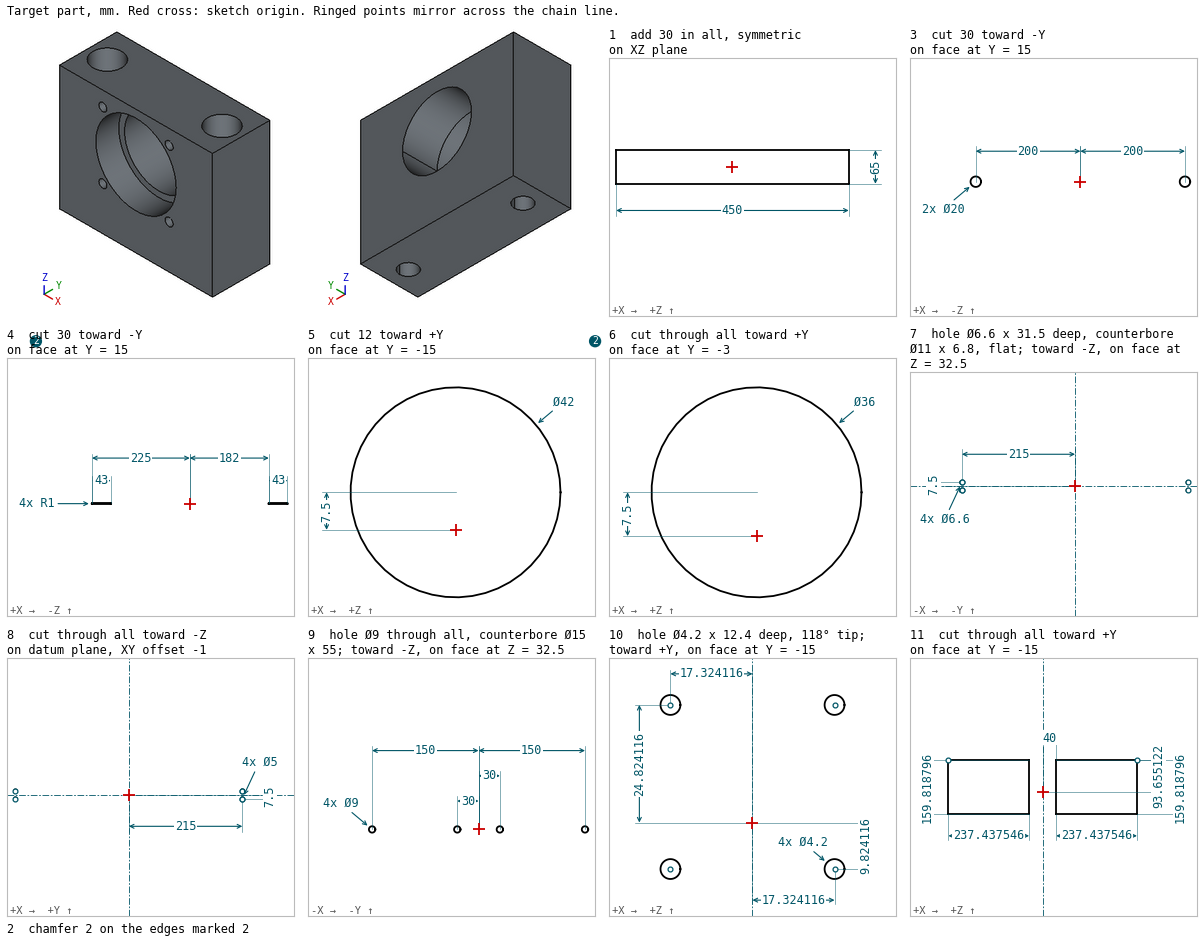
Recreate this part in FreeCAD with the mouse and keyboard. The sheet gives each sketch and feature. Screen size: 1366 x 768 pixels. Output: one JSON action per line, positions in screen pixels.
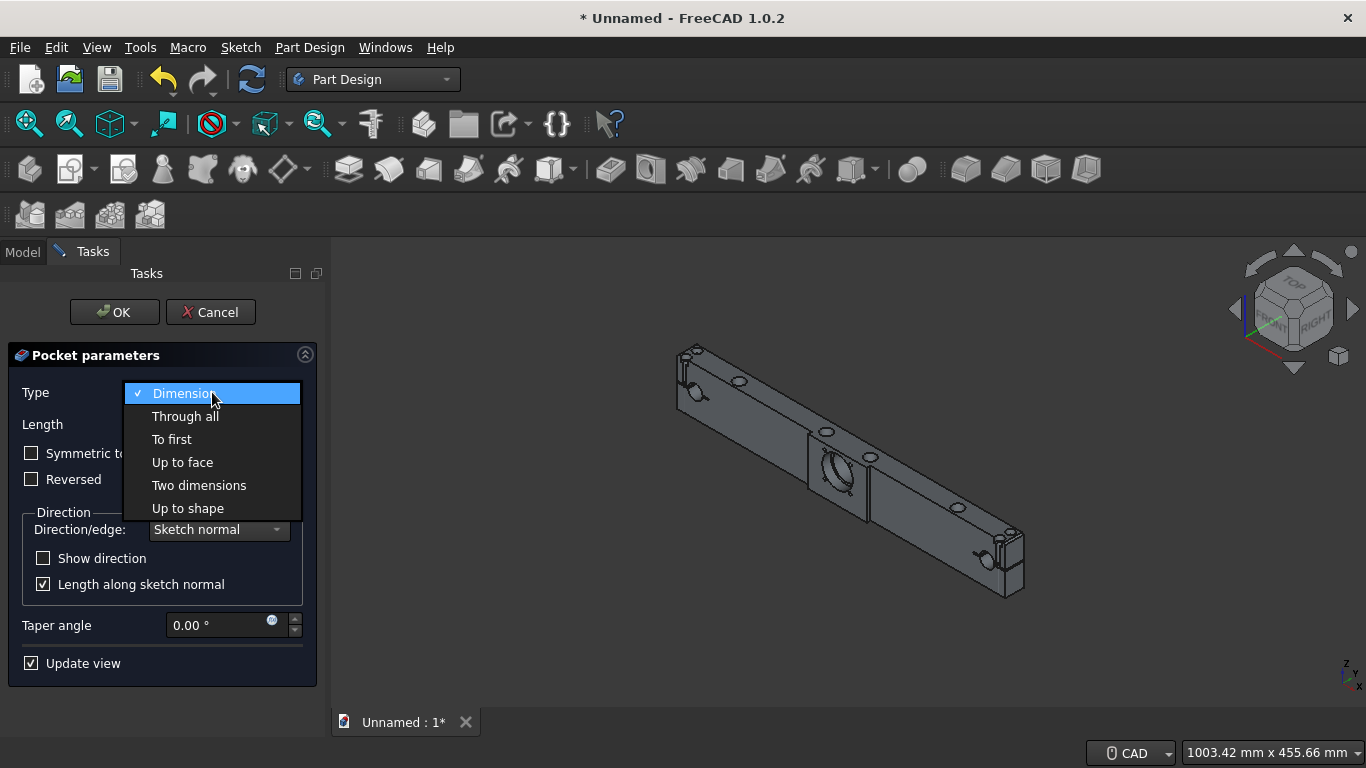
{"action": "left_click", "coordinate": [212, 416]}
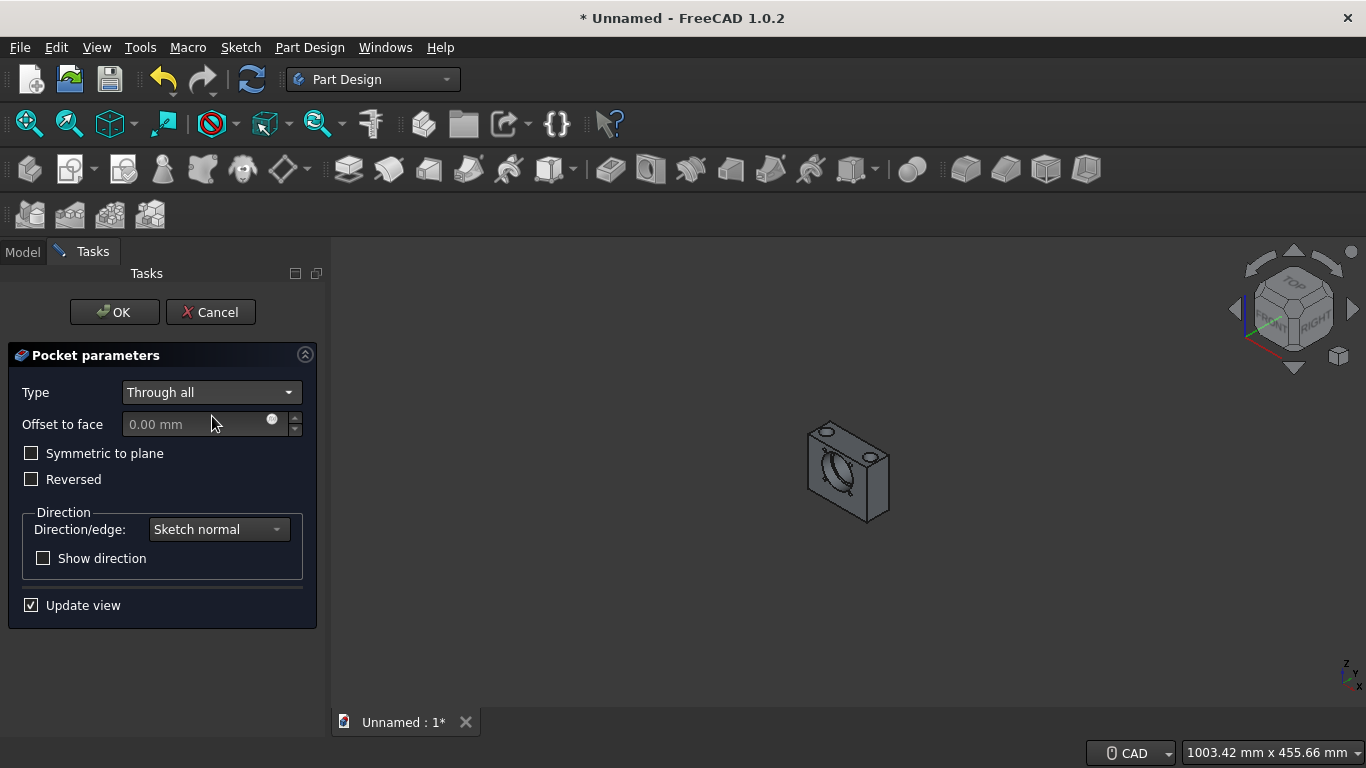
{"action": "left_click", "coordinate": [115, 312]}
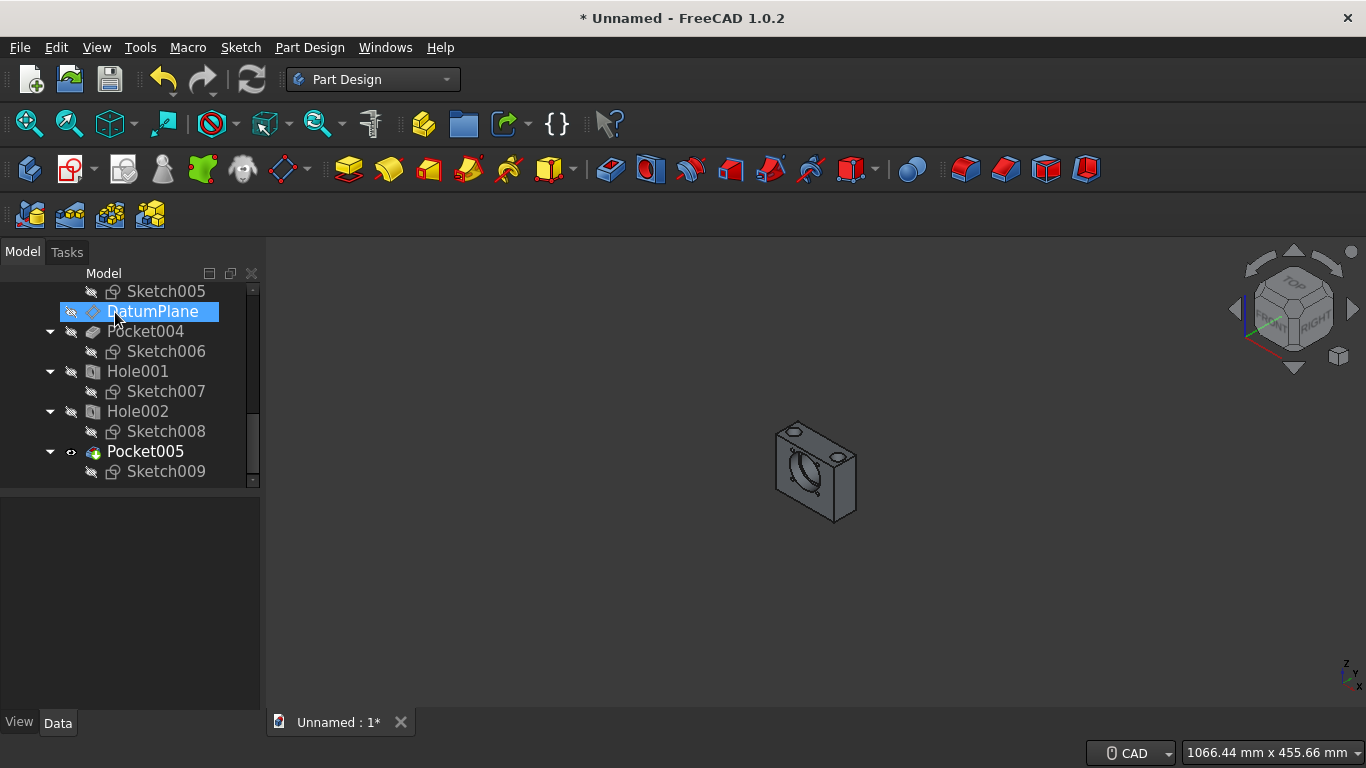
{"action": "left_click", "coordinate": [30, 124]}